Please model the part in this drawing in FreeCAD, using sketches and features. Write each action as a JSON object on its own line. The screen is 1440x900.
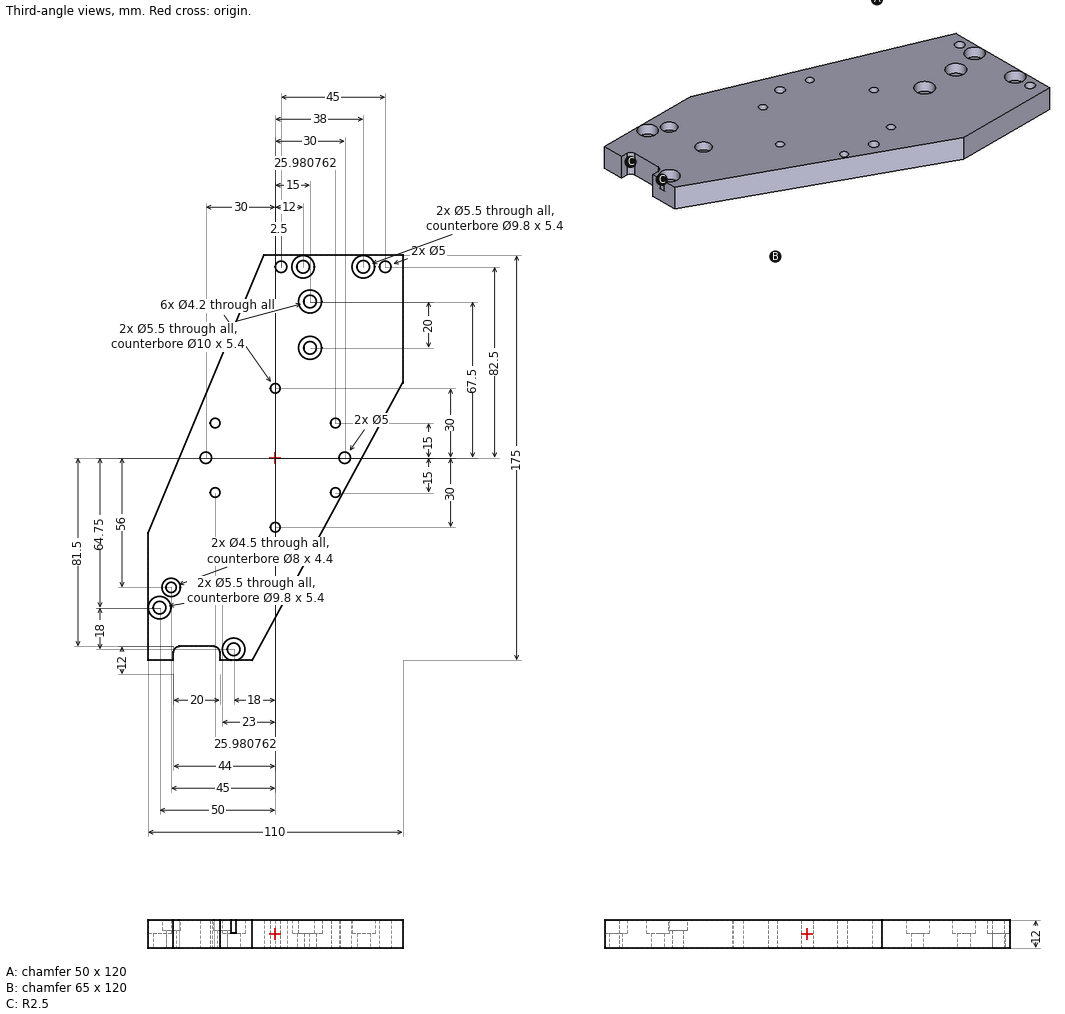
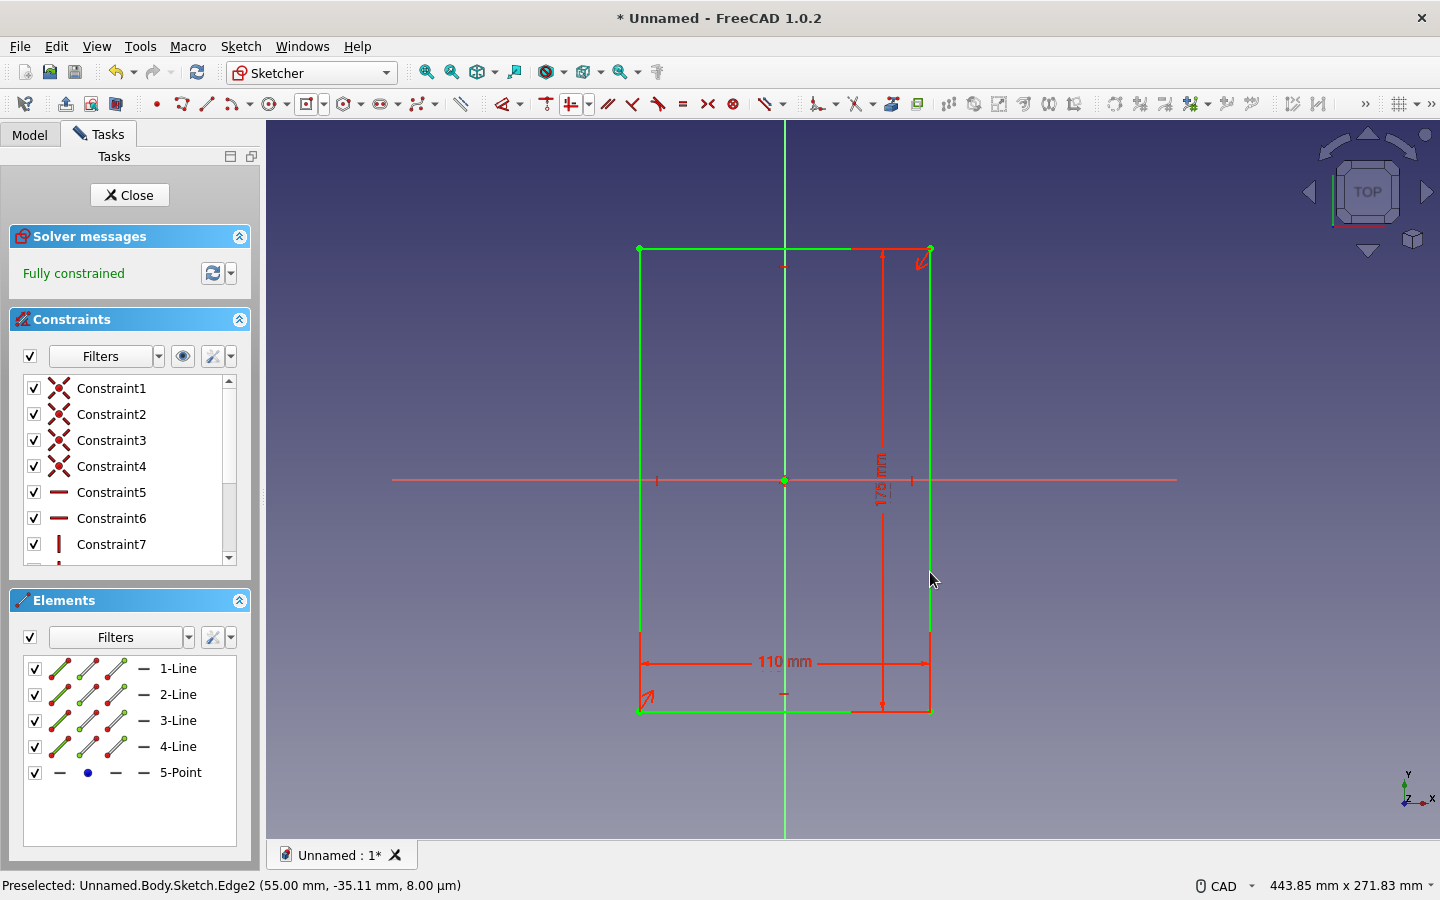
{"action": "left_click", "coordinate": [130, 195]}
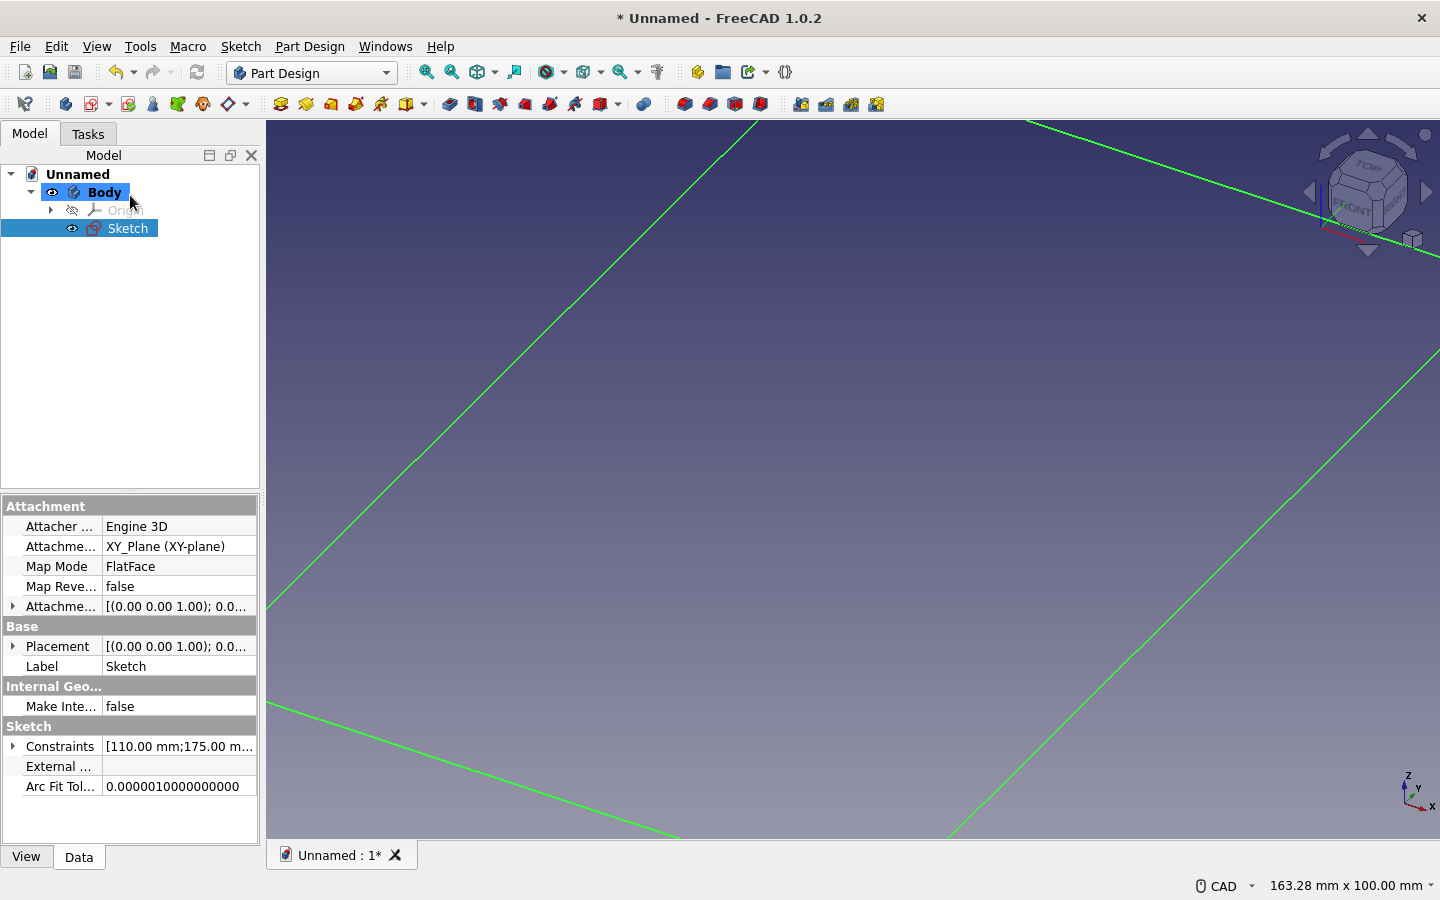
{"action": "left_click", "coordinate": [281, 104]}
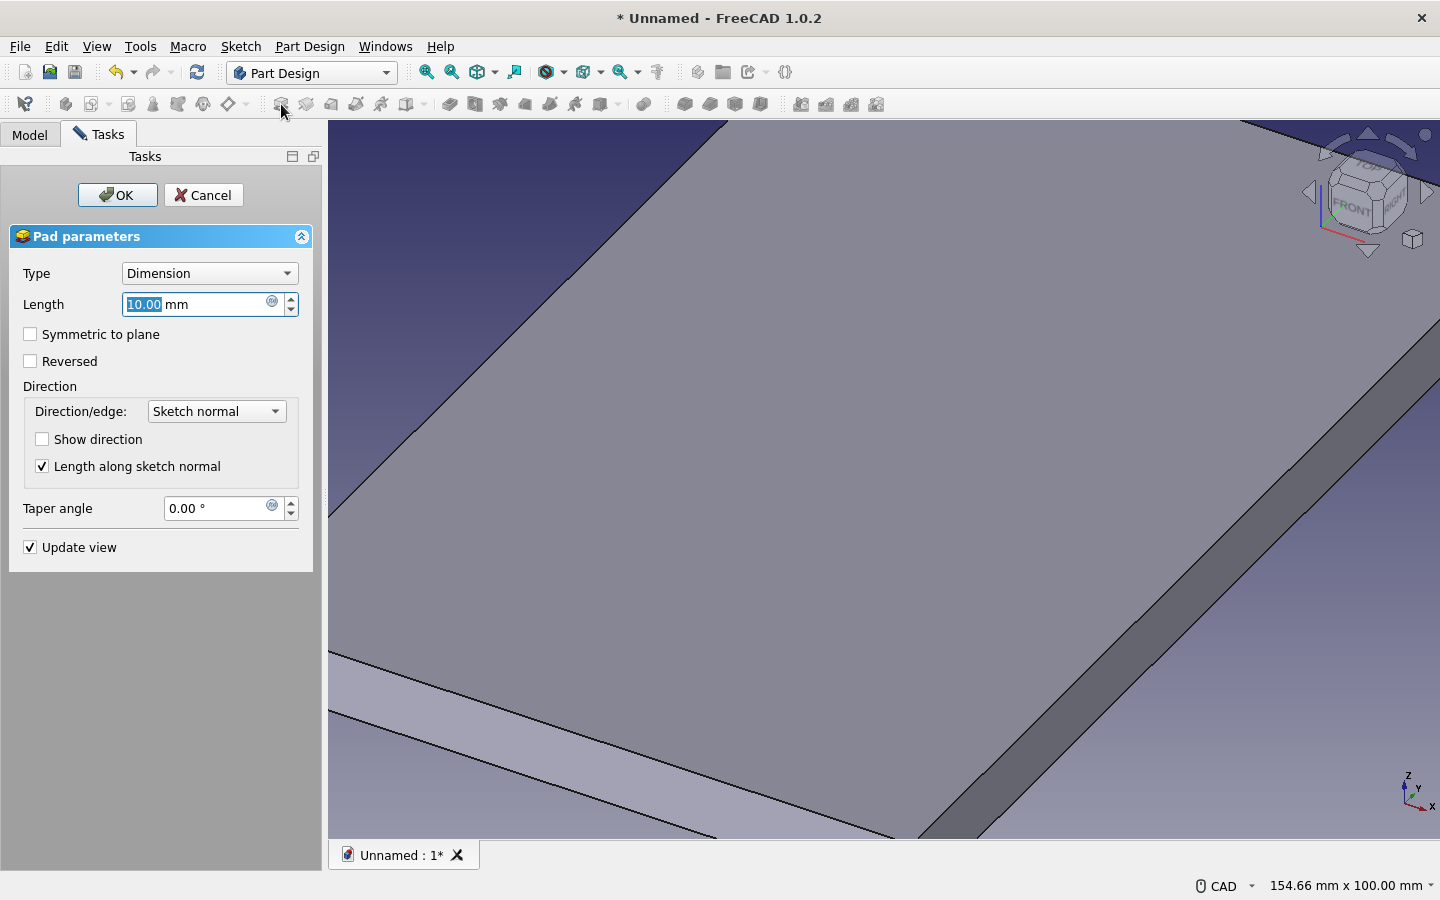
{"action": "type", "text": "12"}
{"action": "key", "text": "Tab"}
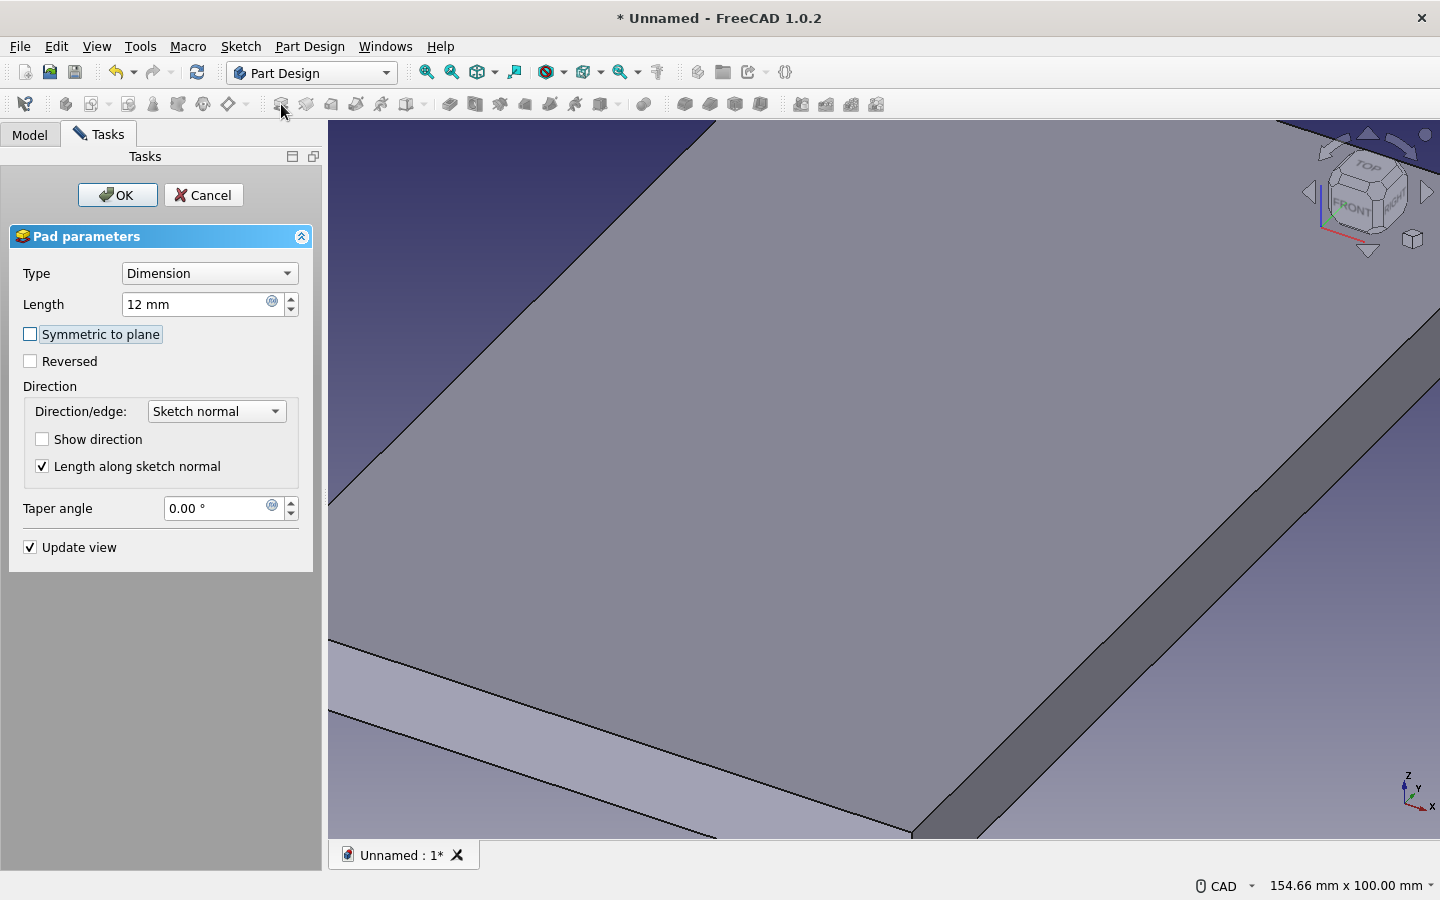
{"action": "left_click", "coordinate": [31, 334]}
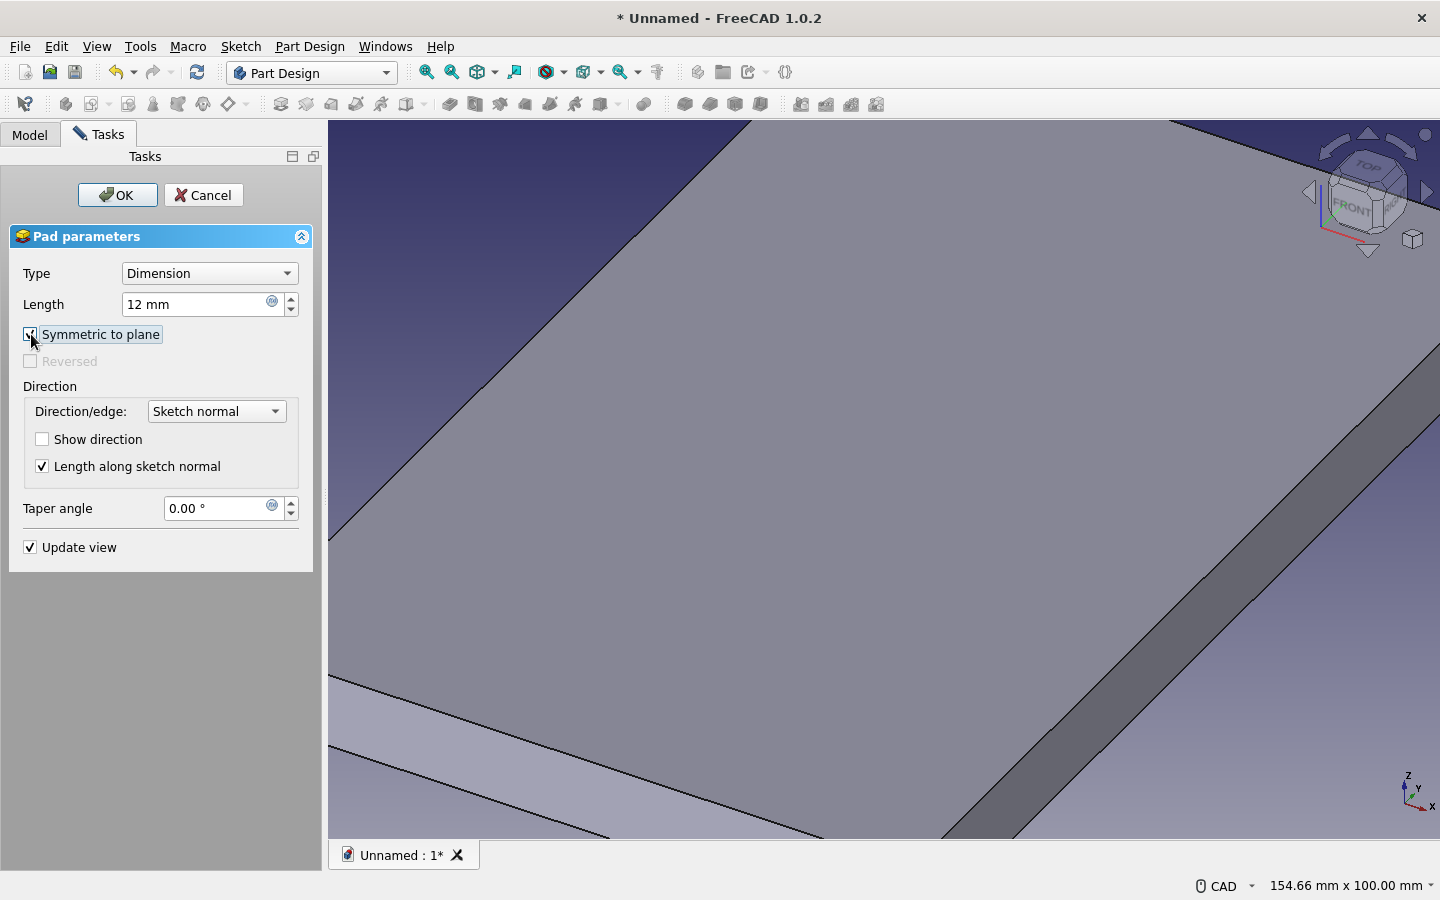
{"action": "left_click", "coordinate": [118, 195]}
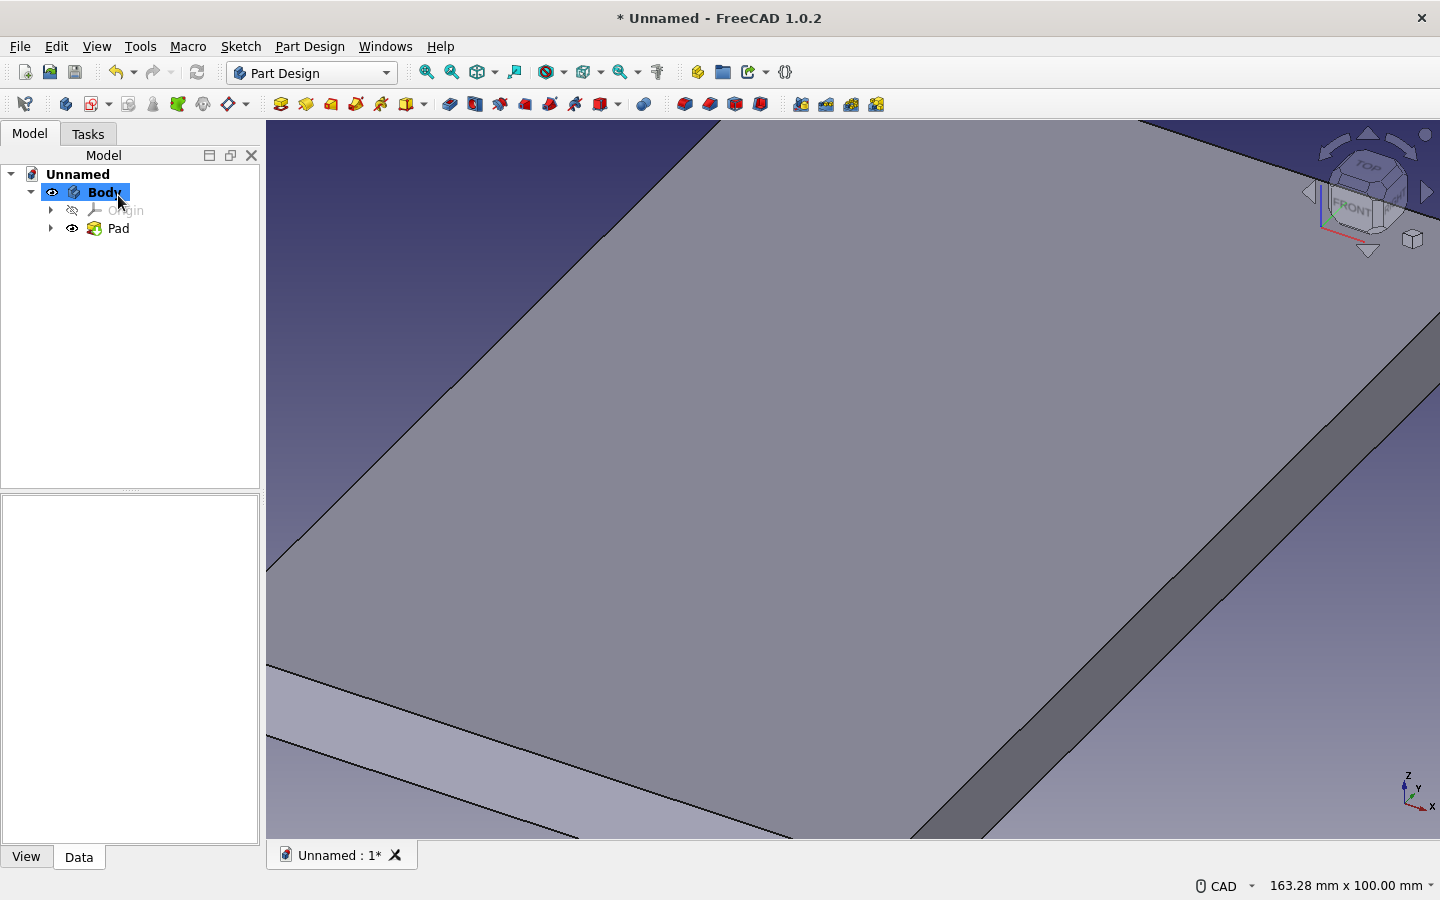
{"action": "key", "text": "v f"}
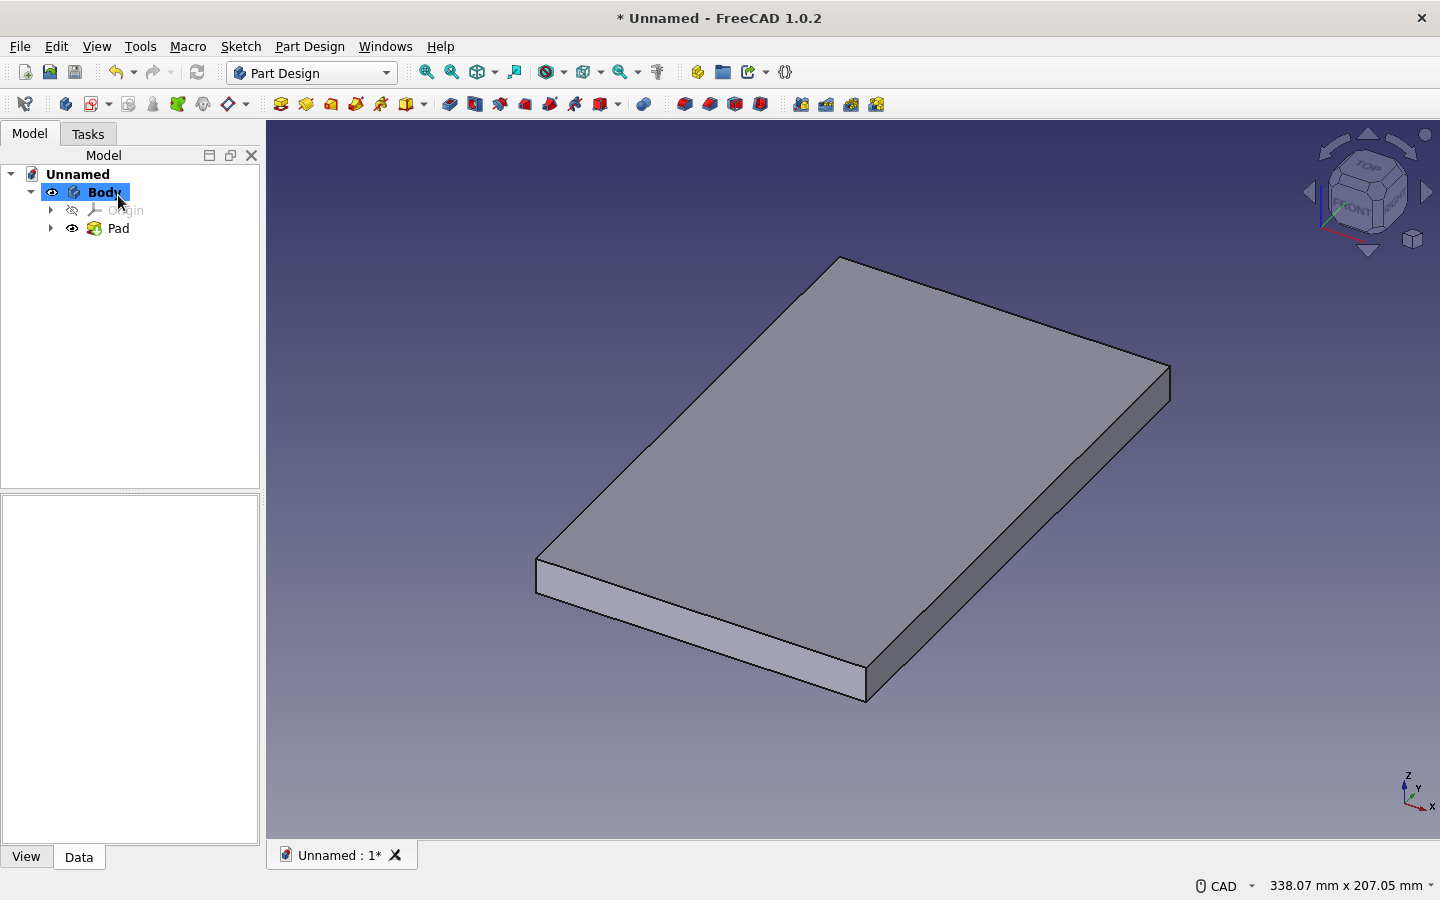
{"action": "key", "text": "0"}